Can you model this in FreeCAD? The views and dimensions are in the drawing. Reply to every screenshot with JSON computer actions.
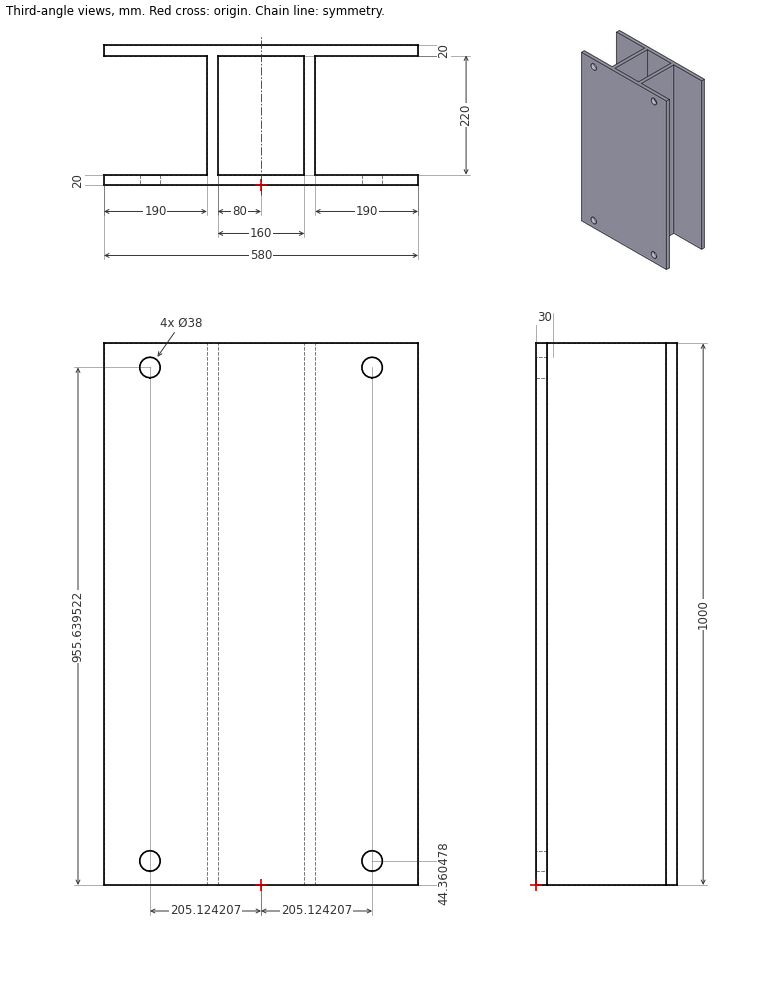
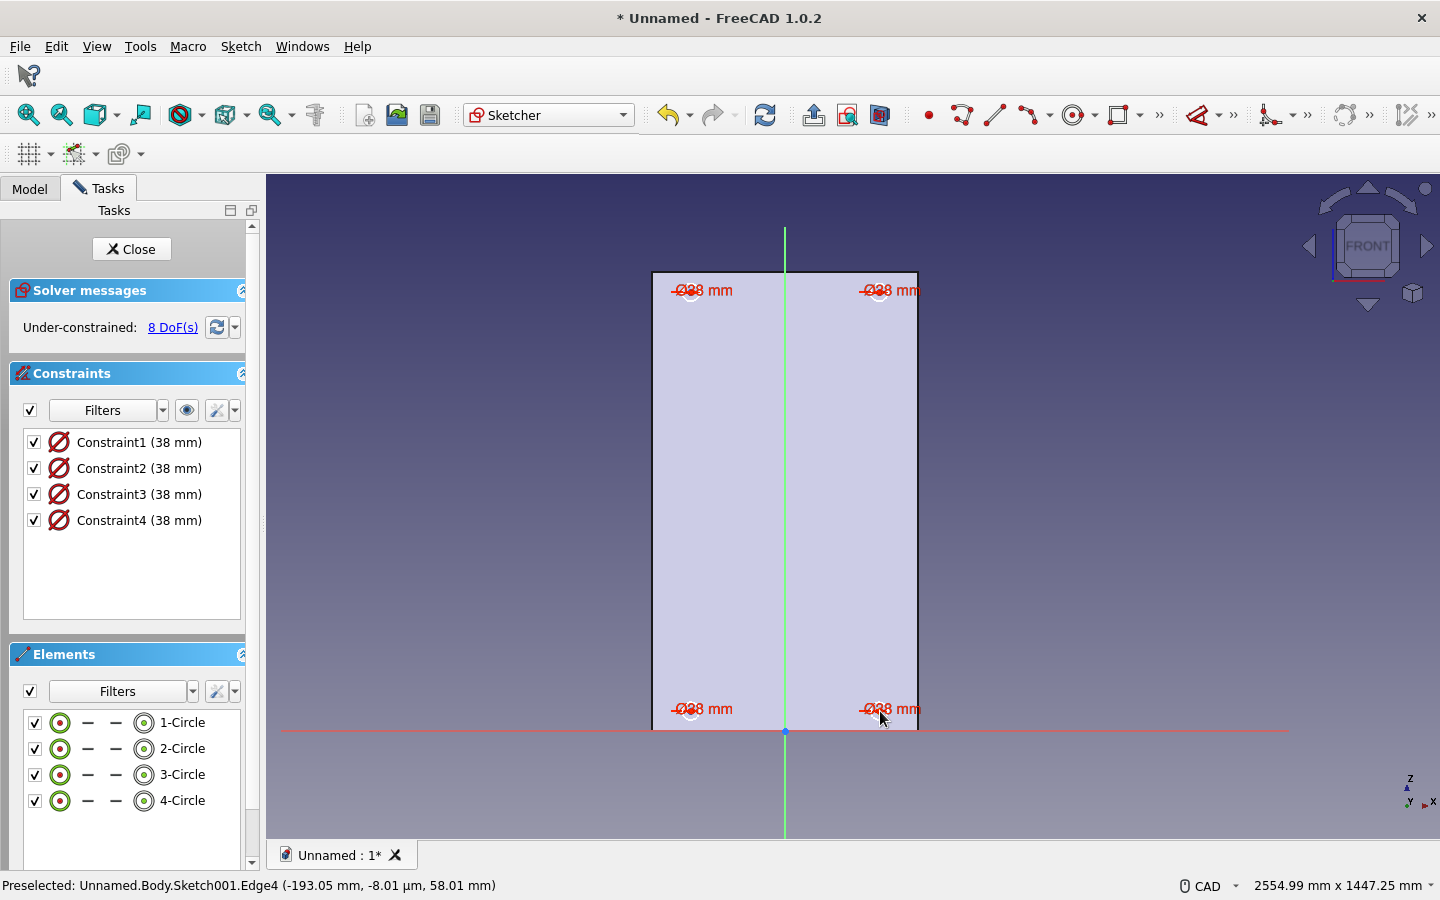
{"action": "left_click", "coordinate": [691, 292]}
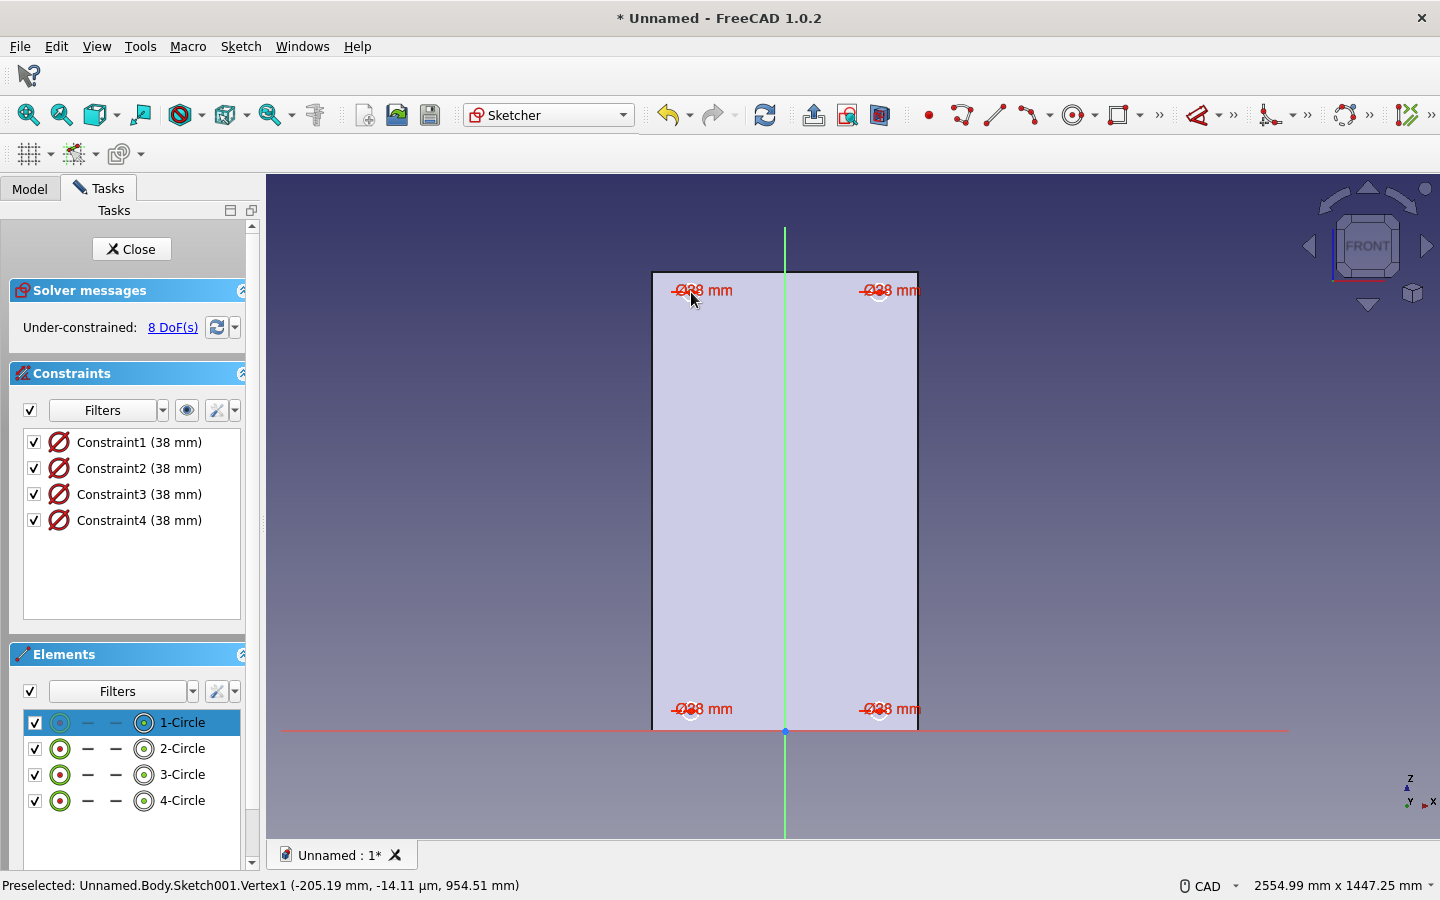
{"action": "left_click", "coordinate": [879, 292]}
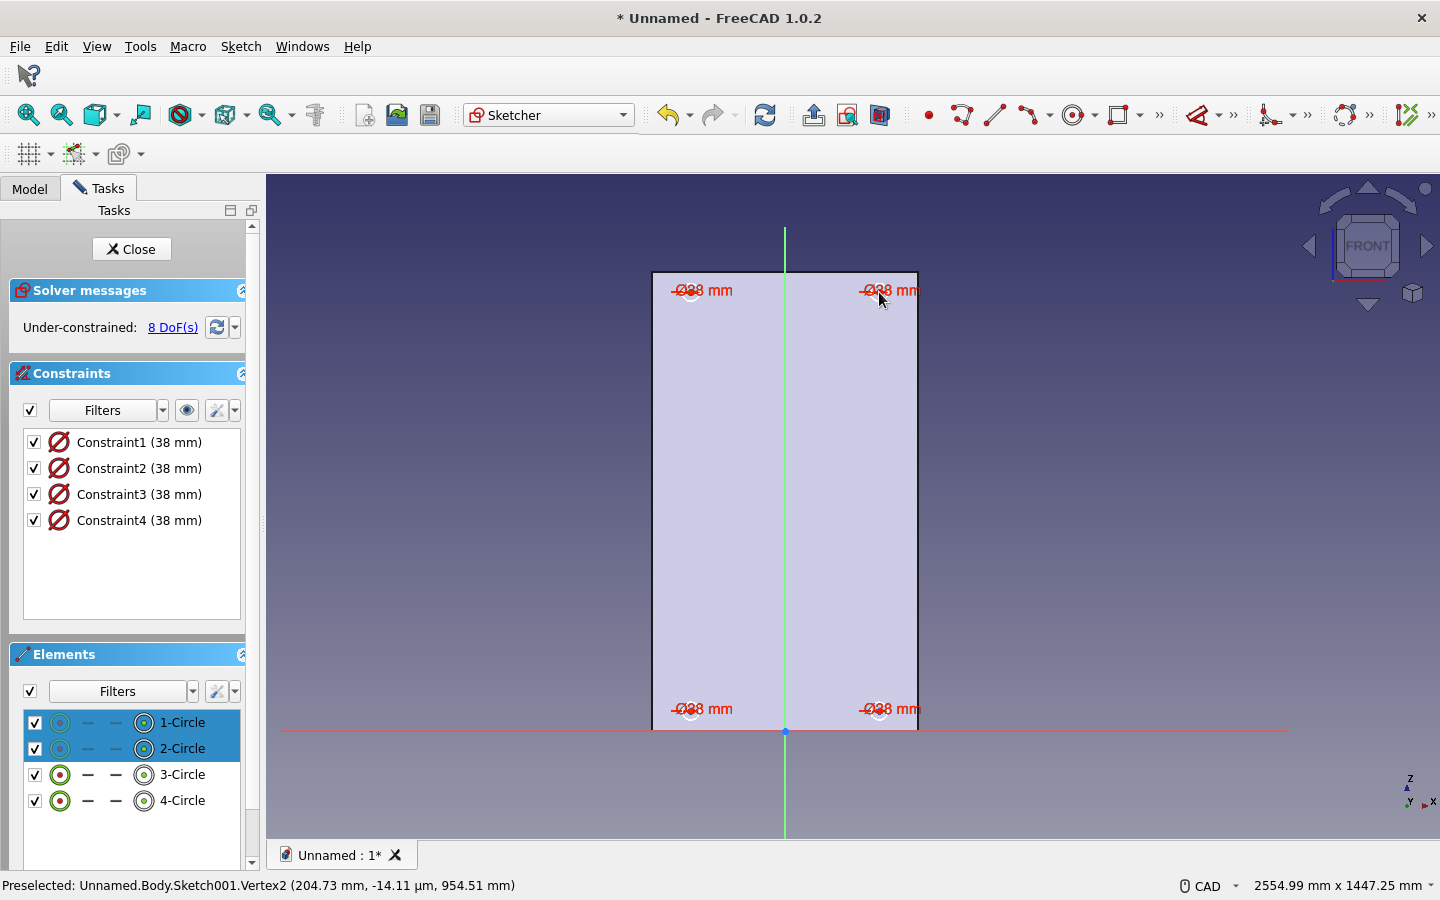
{"action": "key", "text": "h"}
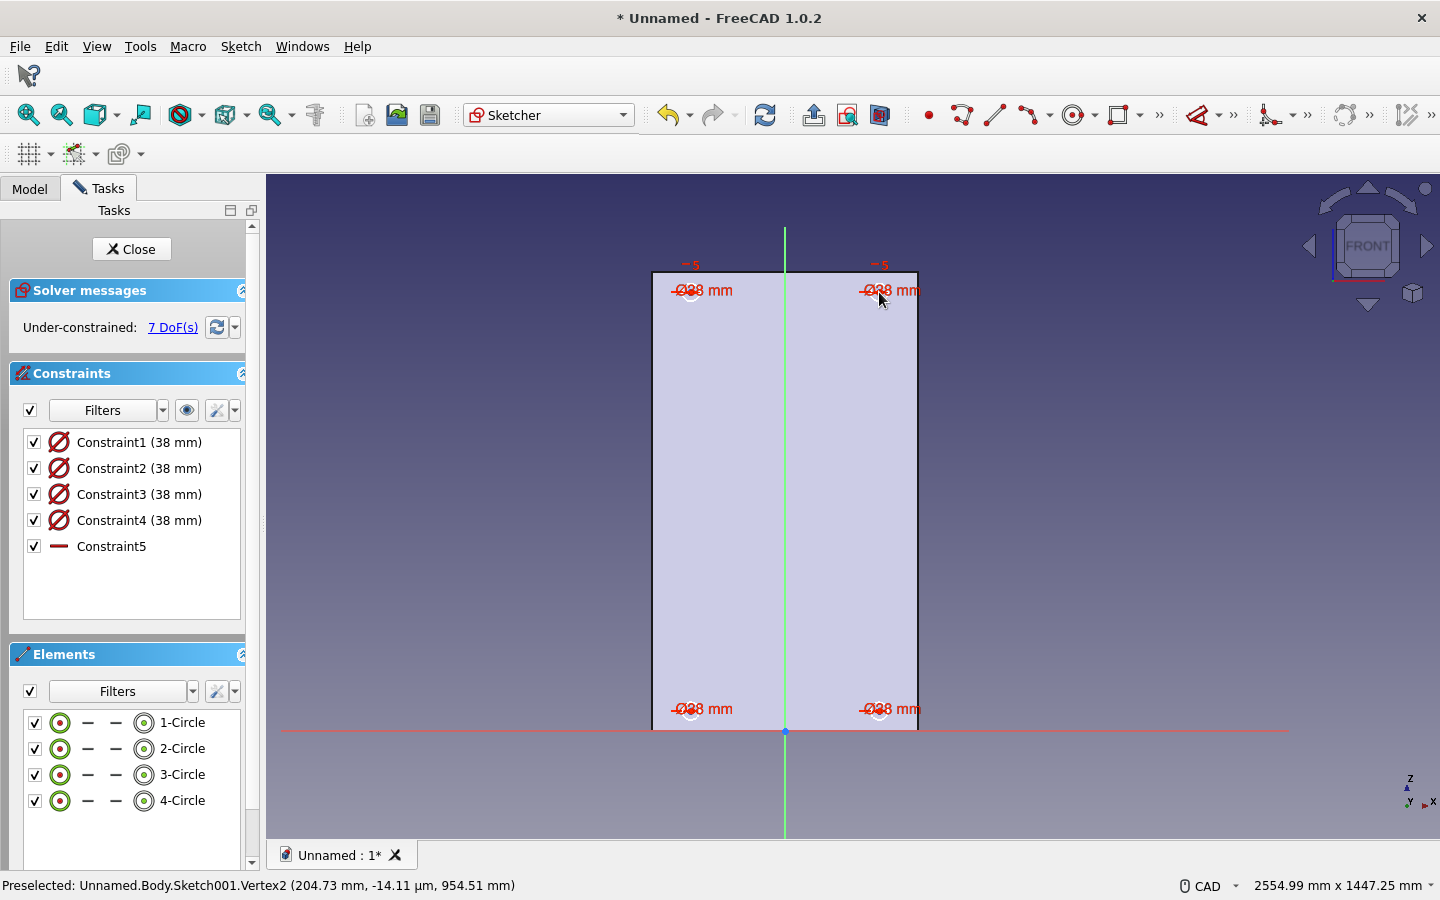
{"action": "left_click", "coordinate": [879, 292]}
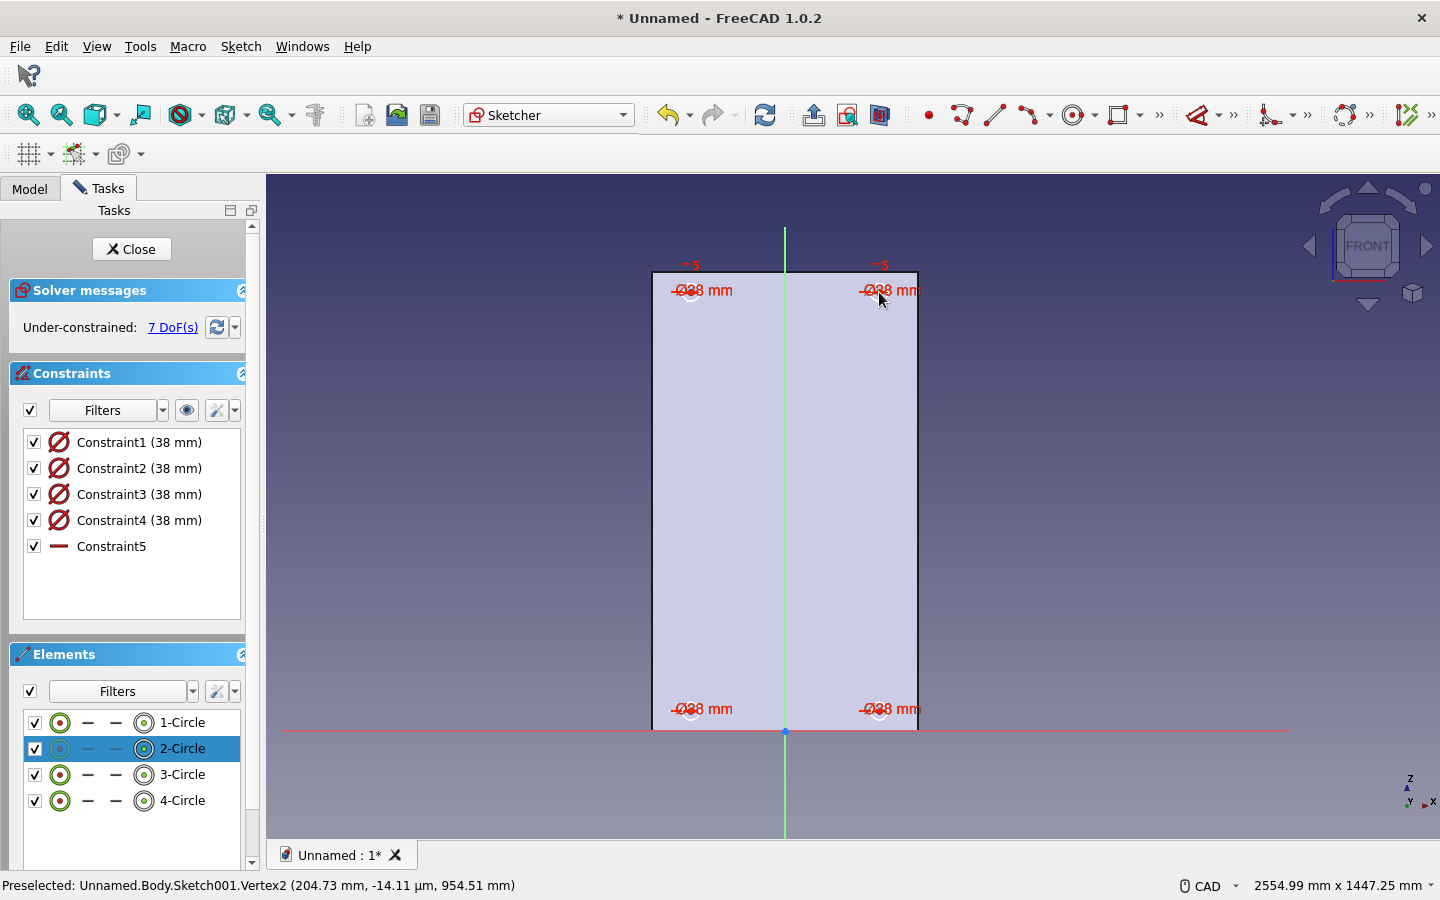
{"action": "left_click", "coordinate": [879, 711]}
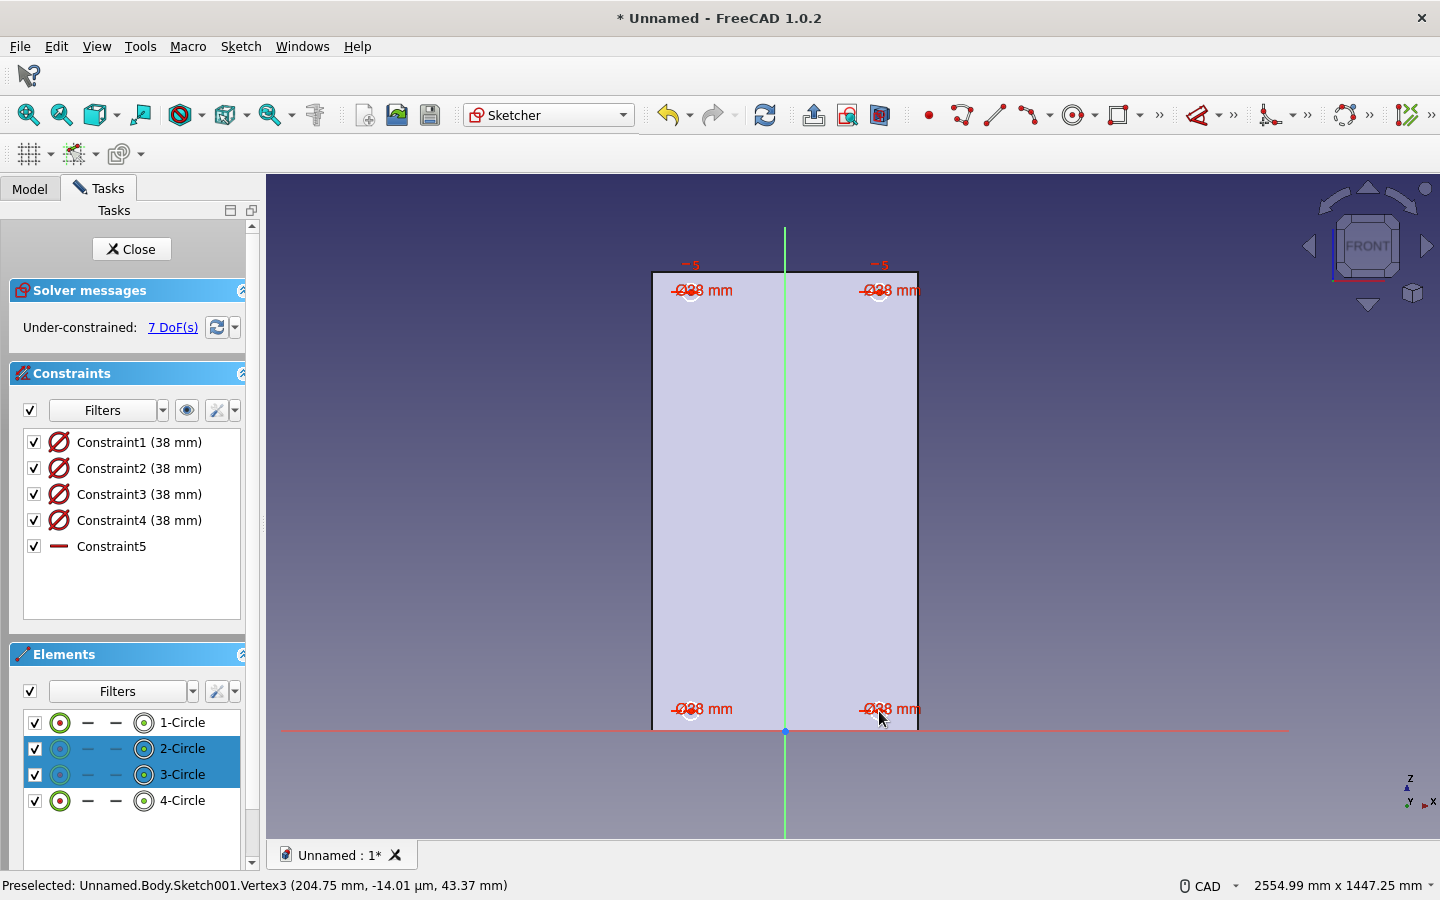
{"action": "key", "text": "v"}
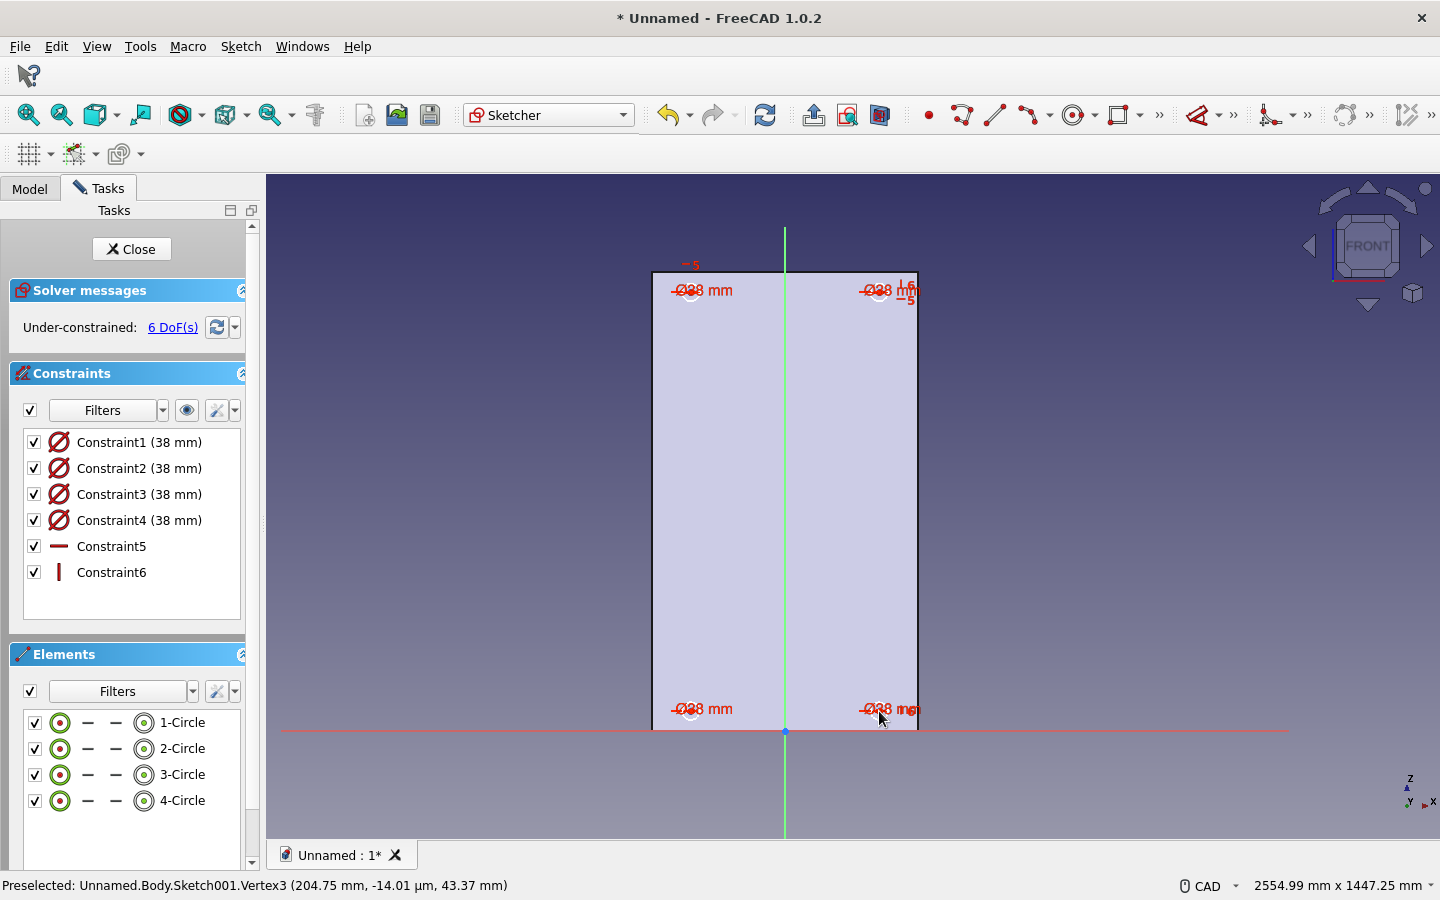
{"action": "left_click", "coordinate": [691, 292]}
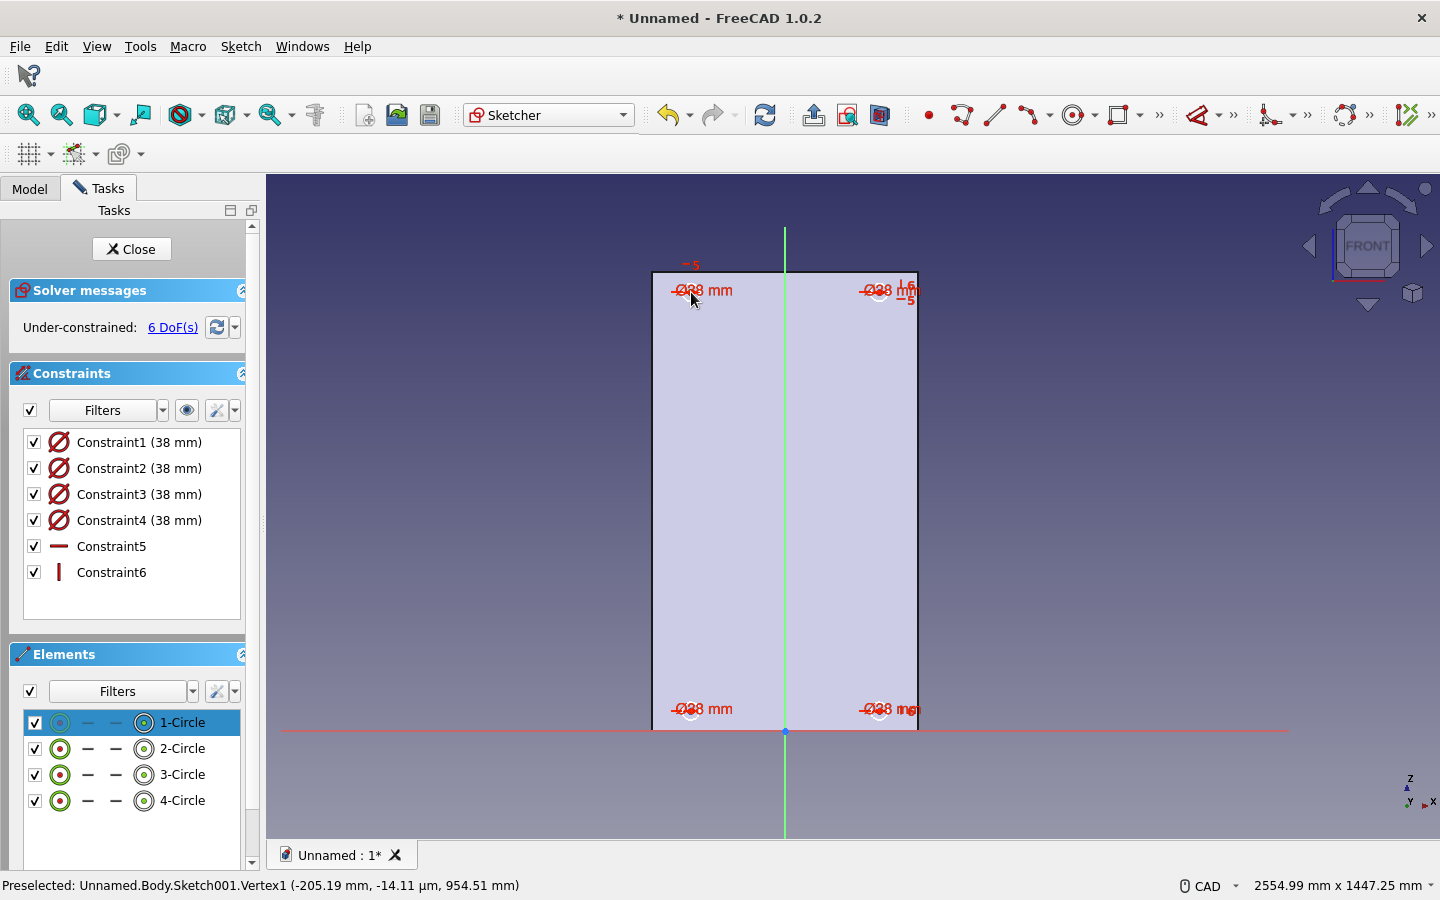
{"action": "left_click", "coordinate": [691, 711]}